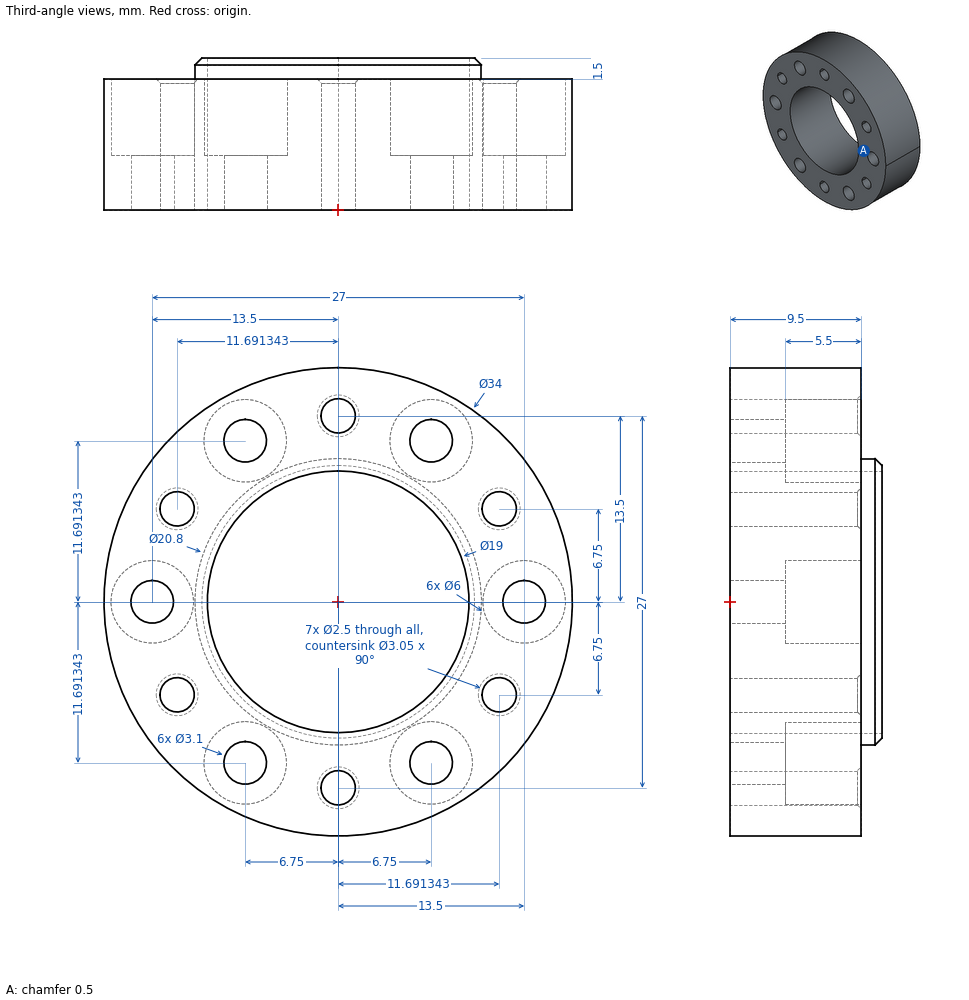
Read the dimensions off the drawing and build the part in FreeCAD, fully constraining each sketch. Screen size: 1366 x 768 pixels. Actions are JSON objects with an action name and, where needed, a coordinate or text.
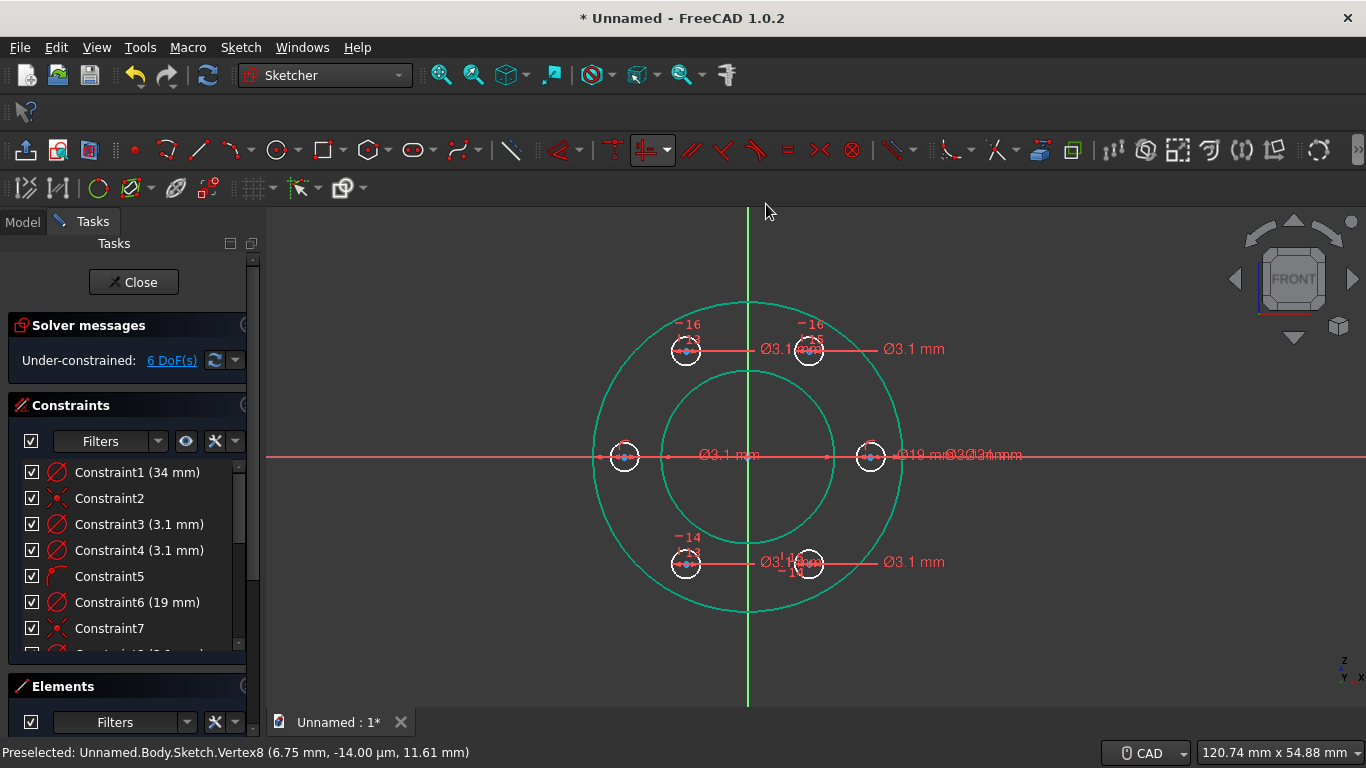
{"action": "left_click", "coordinate": [558, 150]}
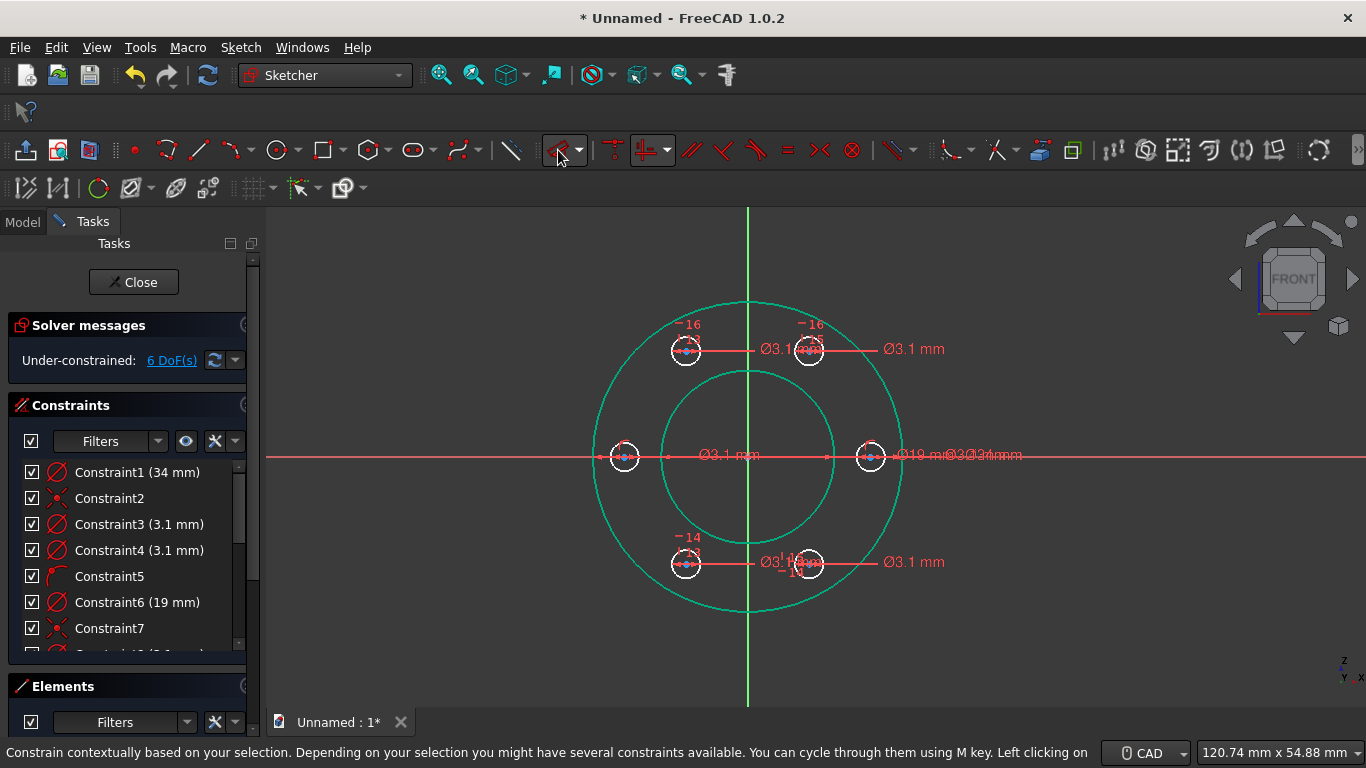
{"action": "left_click", "coordinate": [625, 457]}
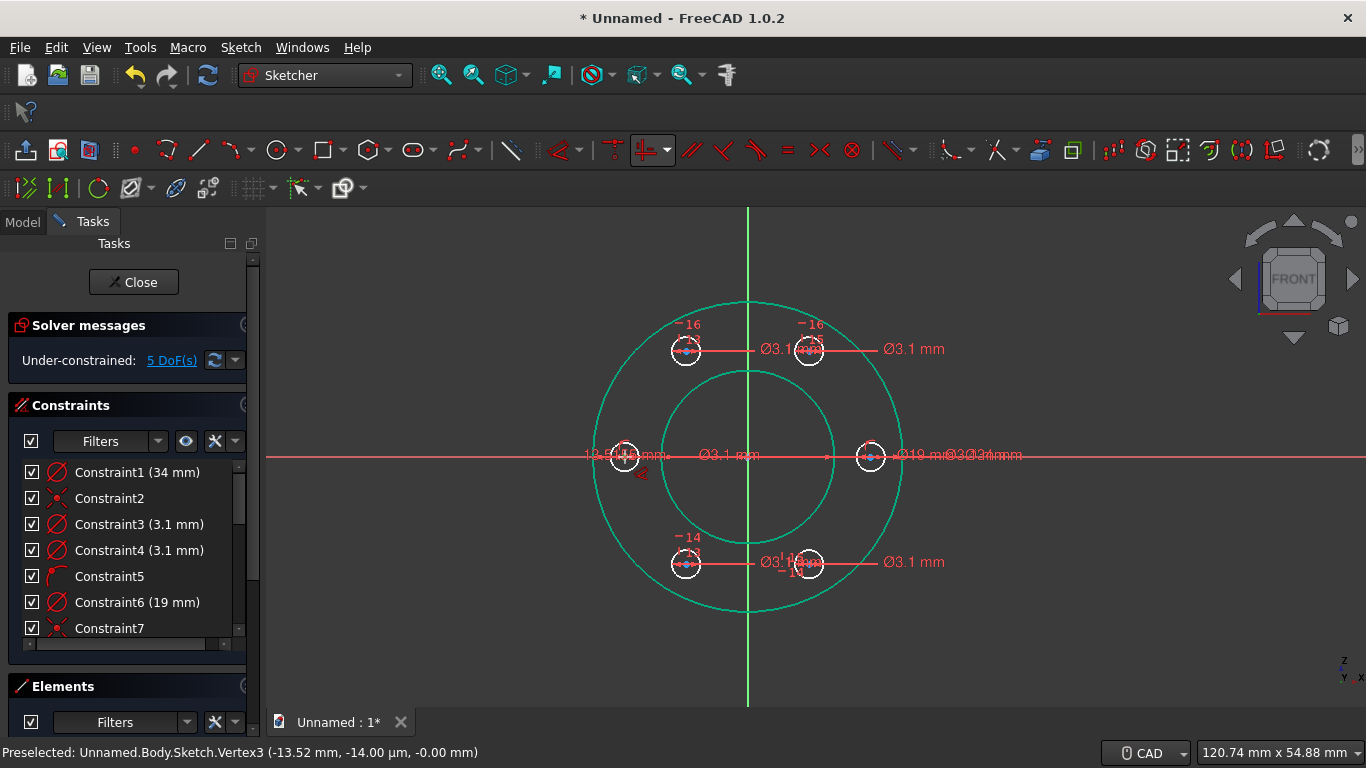
{"action": "left_click", "coordinate": [871, 457]}
{"action": "left_click", "coordinate": [691, 491]}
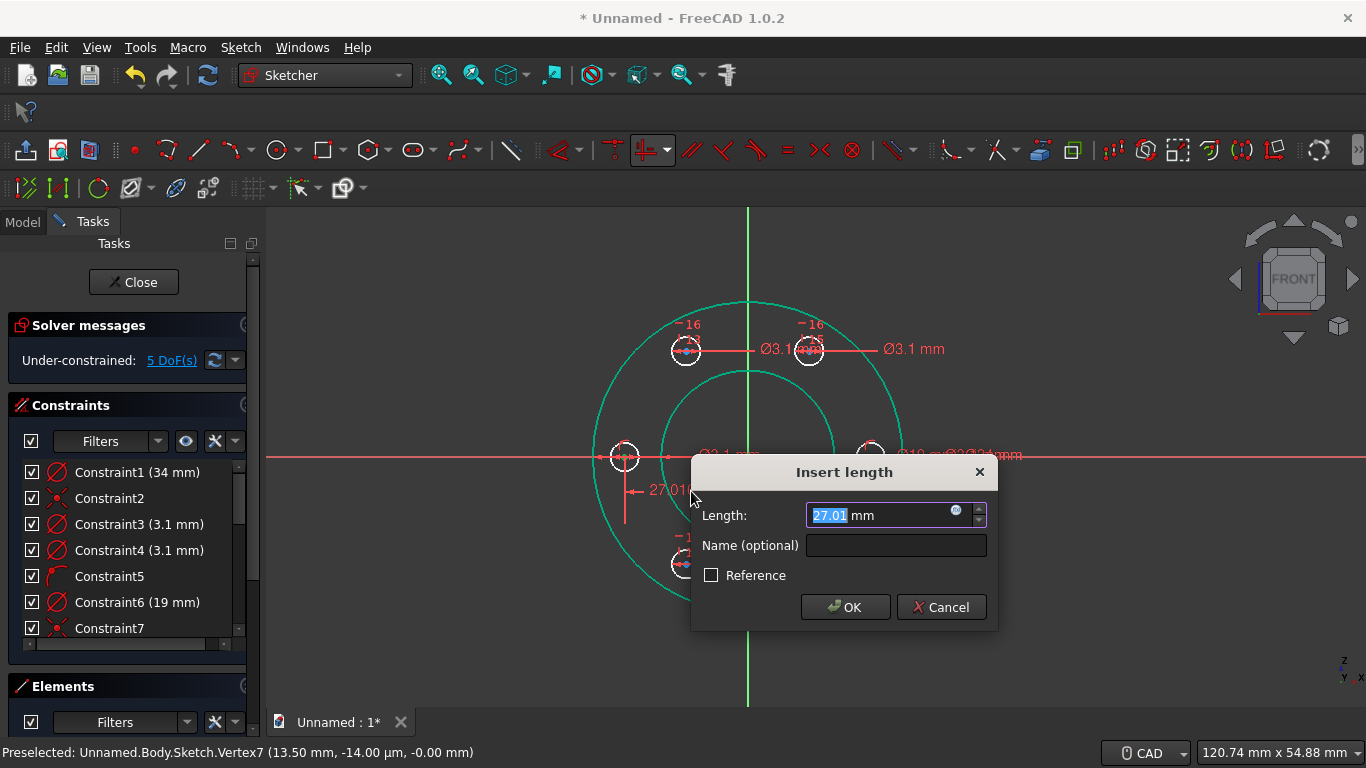
{"action": "type", "text": "27"}
{"action": "key", "text": "Return"}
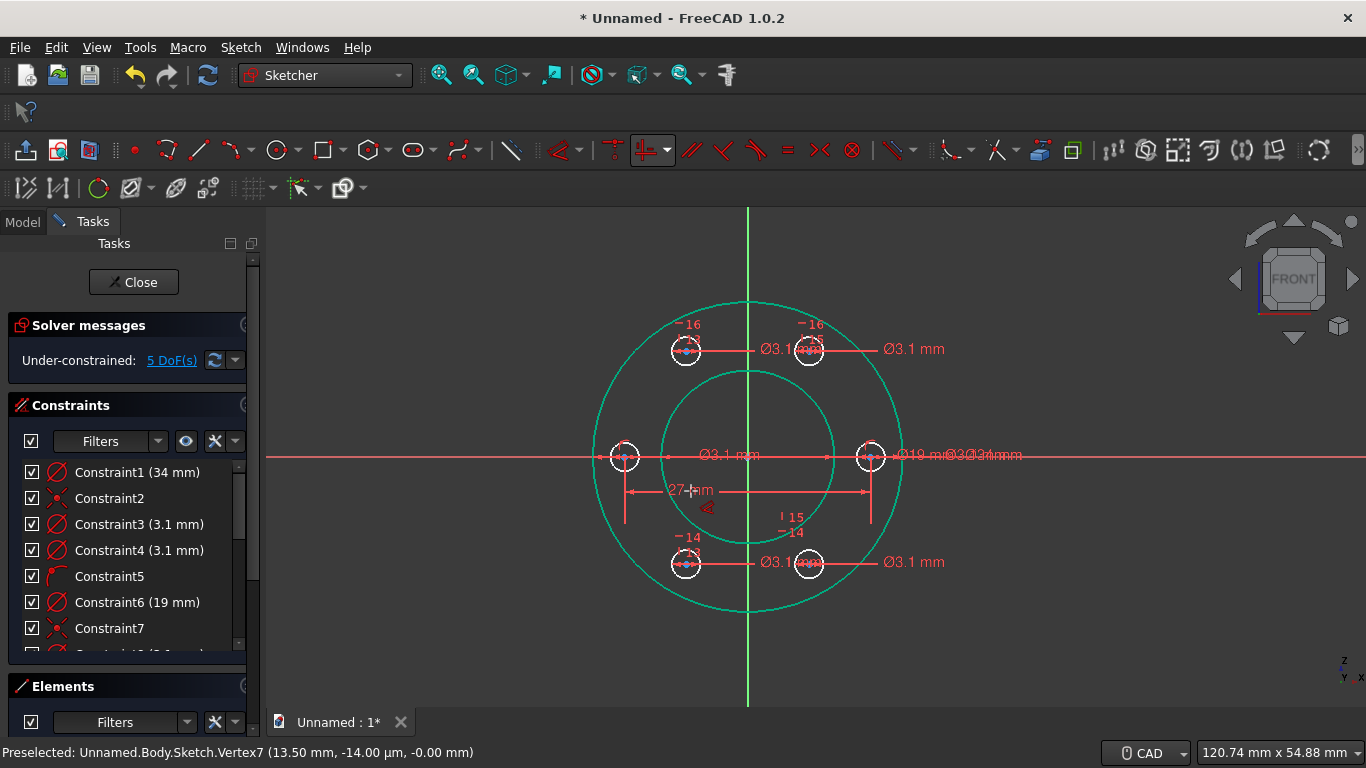
{"action": "left_click", "coordinate": [686, 564]}
{"action": "left_click", "coordinate": [717, 423]}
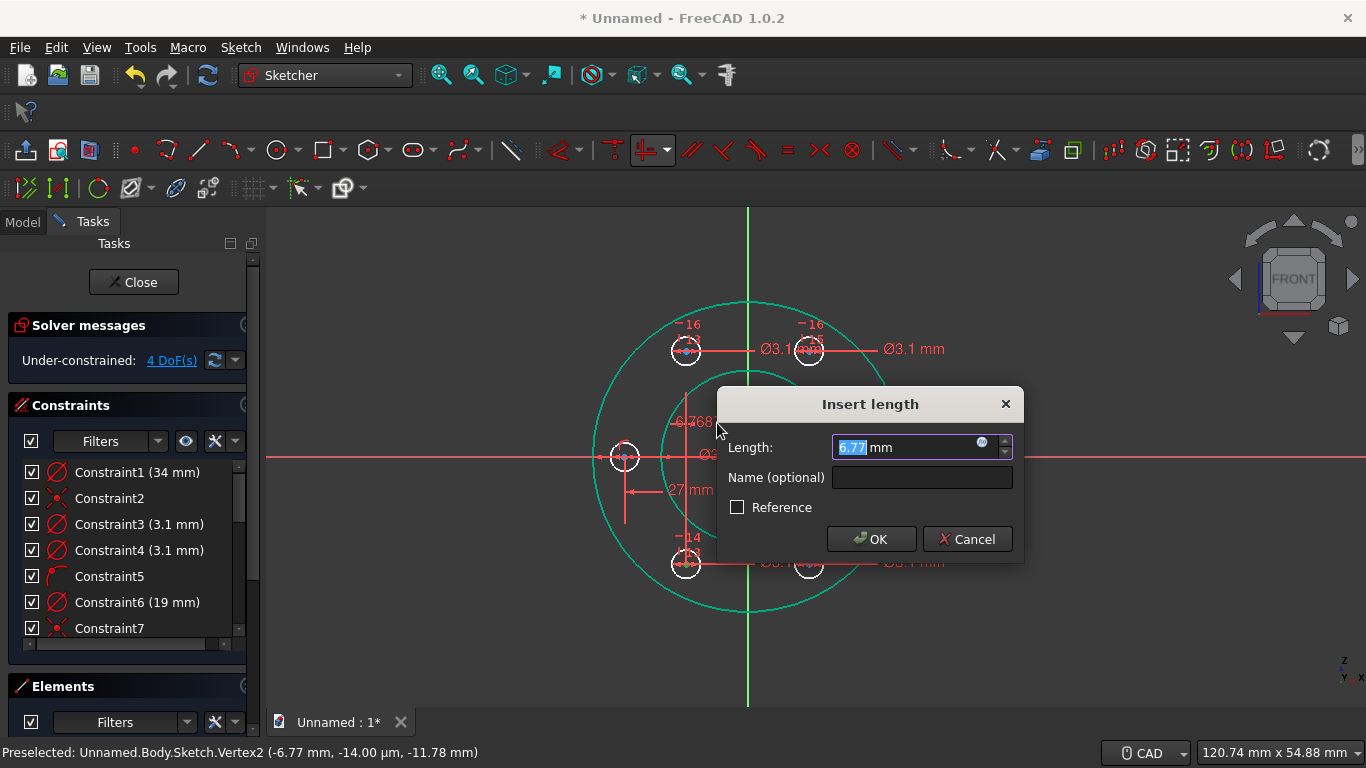
{"action": "type", "text": "6.75"}
{"action": "key", "text": "Return"}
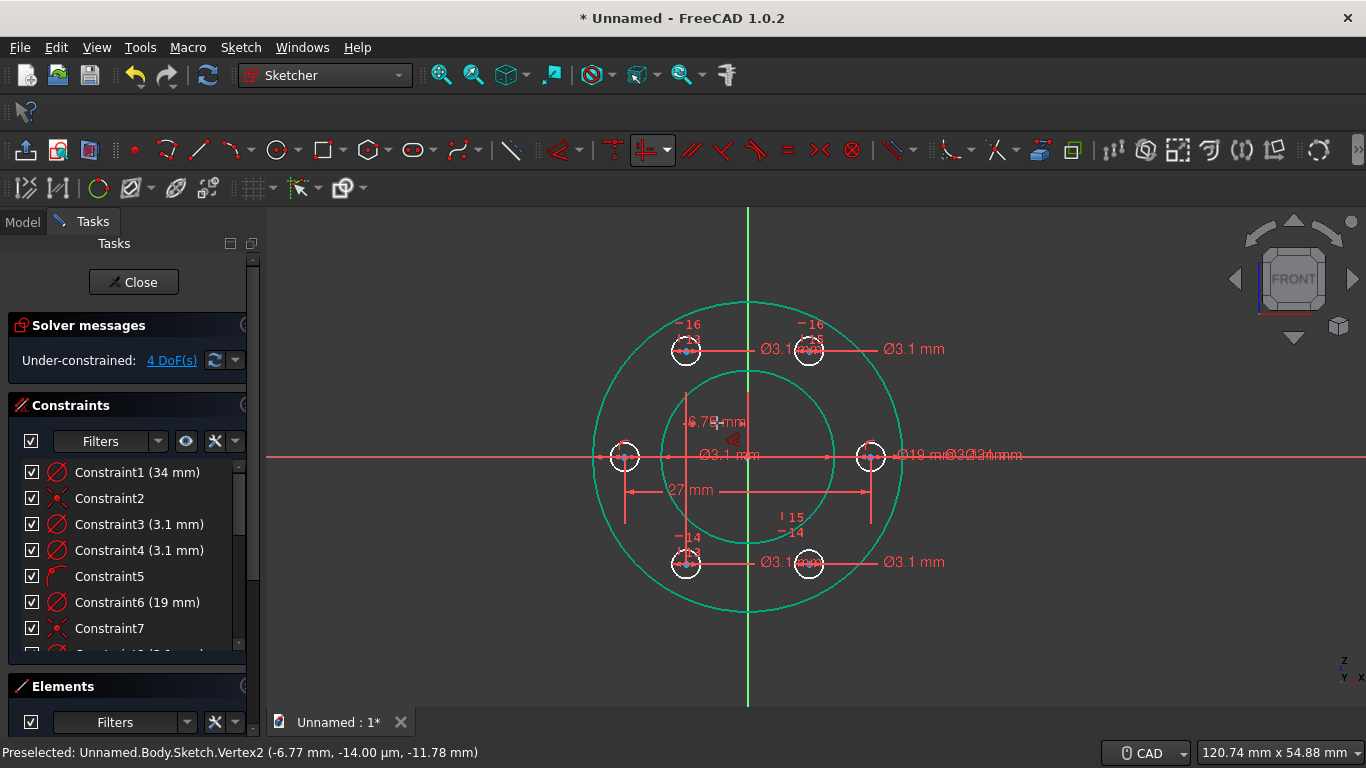
{"action": "left_click", "coordinate": [625, 457]}
{"action": "left_click", "coordinate": [643, 423]}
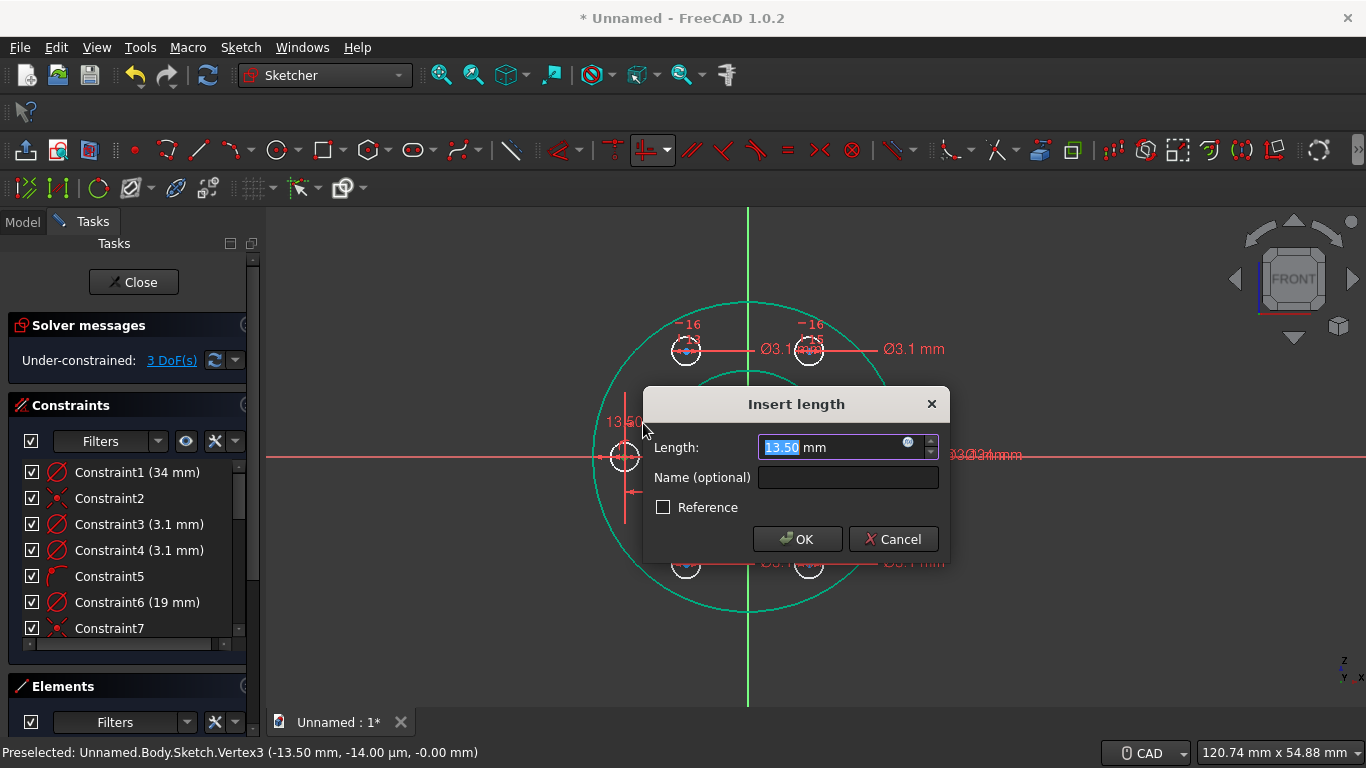
{"action": "type", "text": "13.5"}
{"action": "key", "text": "Return"}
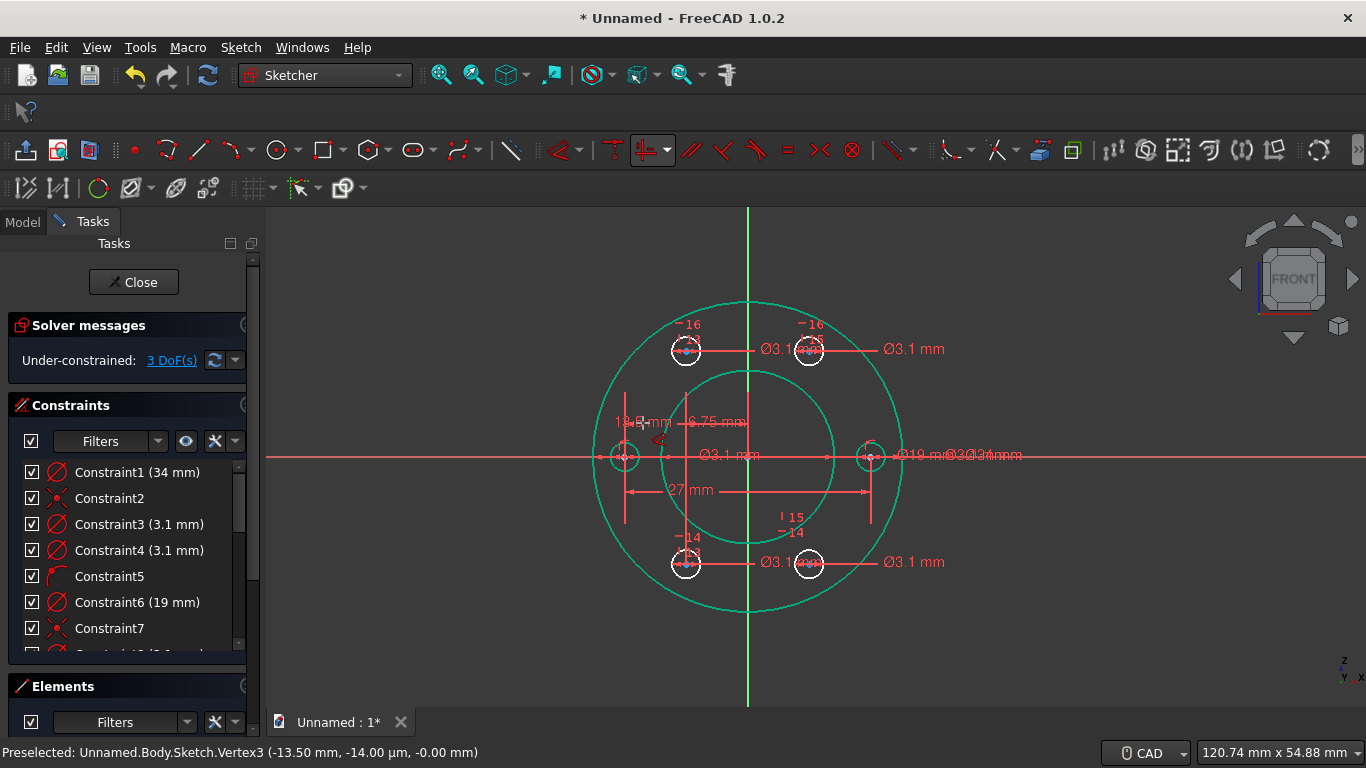
{"action": "left_click", "coordinate": [809, 564]}
{"action": "left_click", "coordinate": [793, 423]}